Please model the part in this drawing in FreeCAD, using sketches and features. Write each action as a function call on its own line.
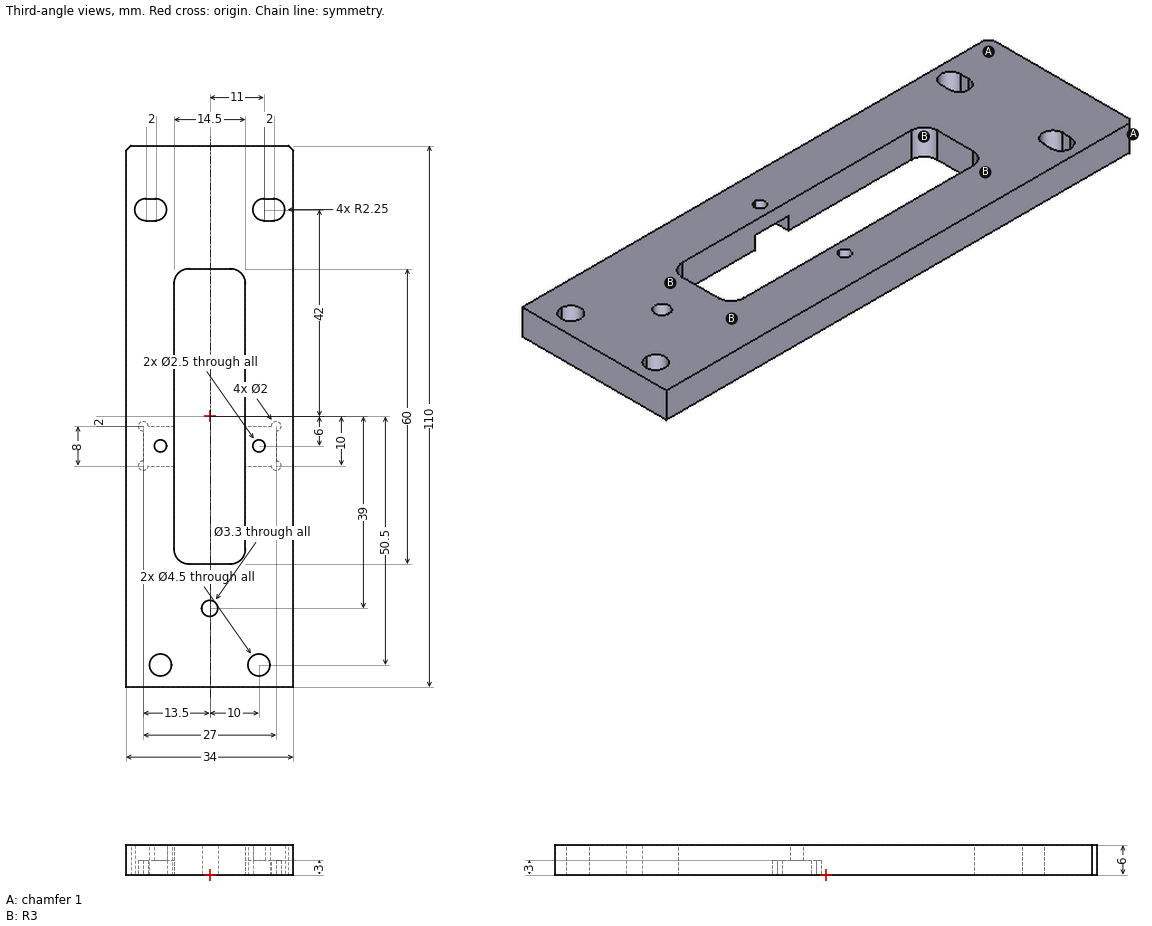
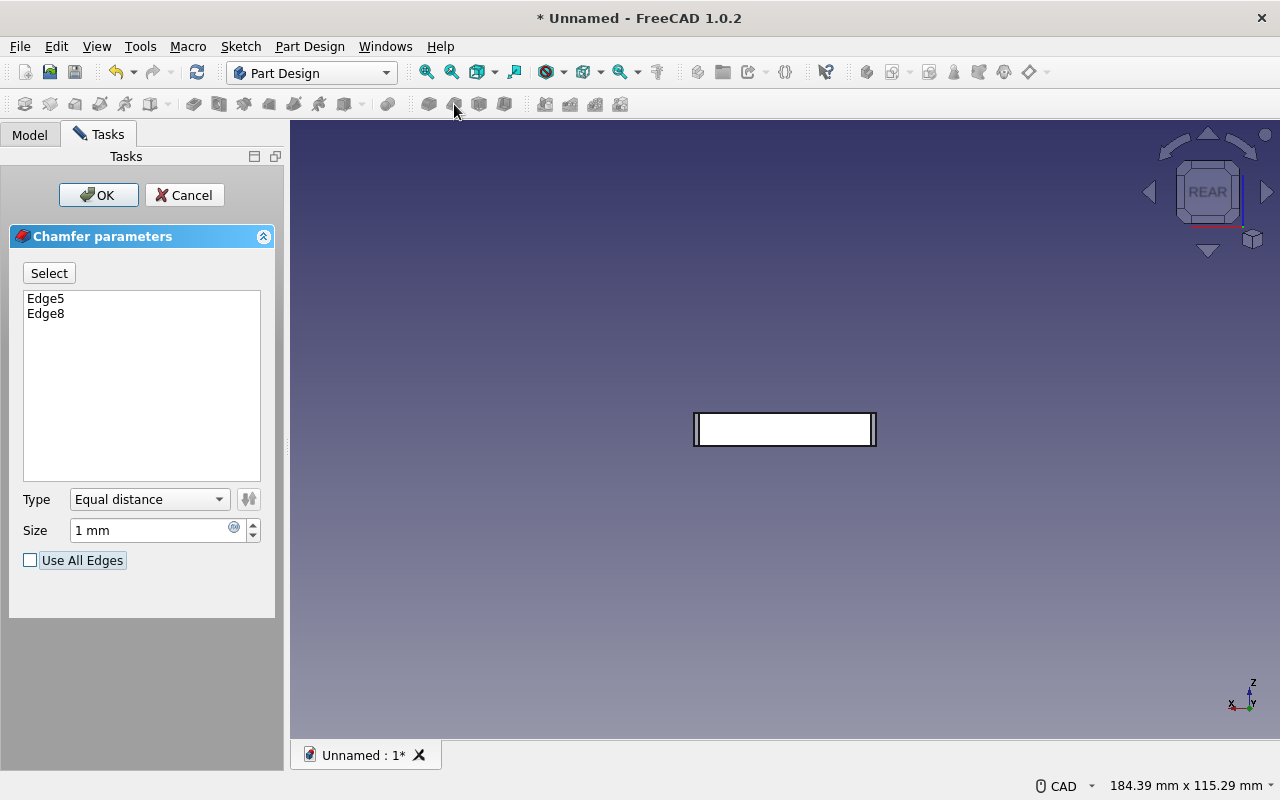
click(99, 195)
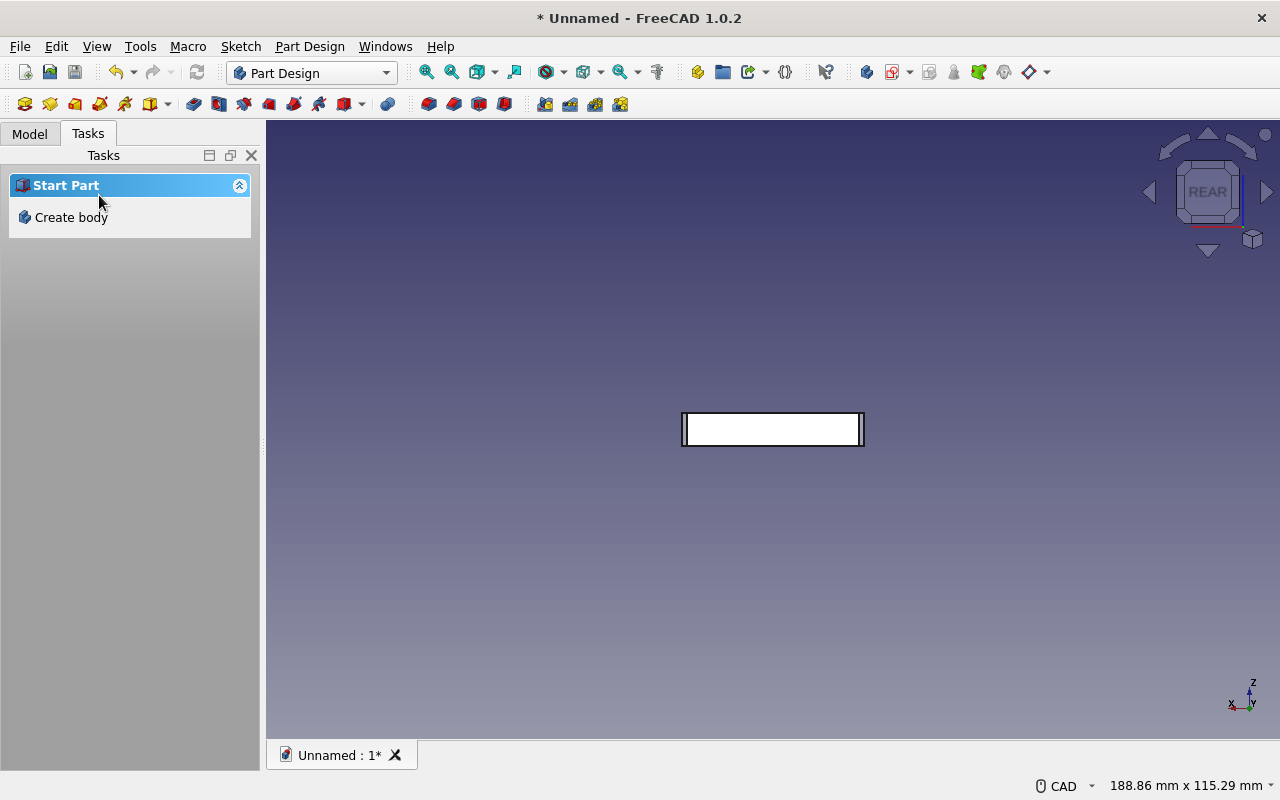
key(v)
key(f)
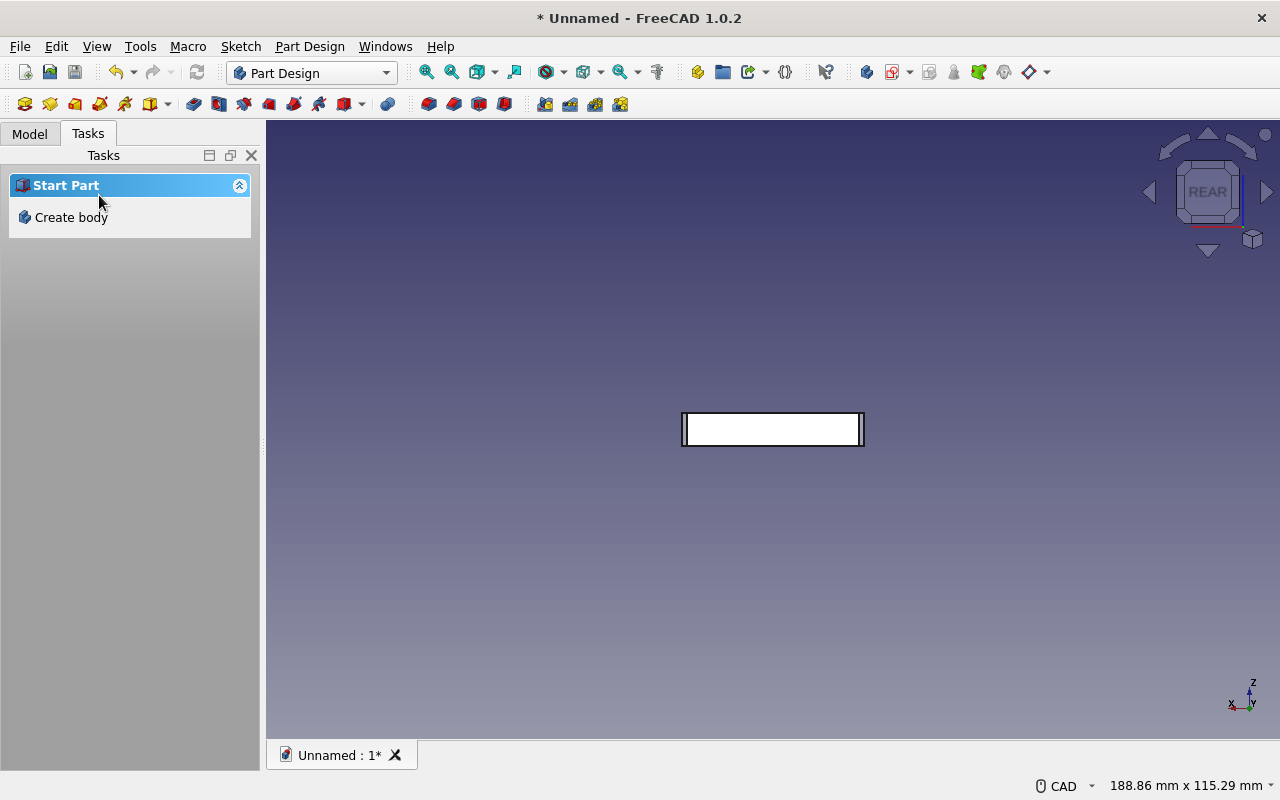
key(5)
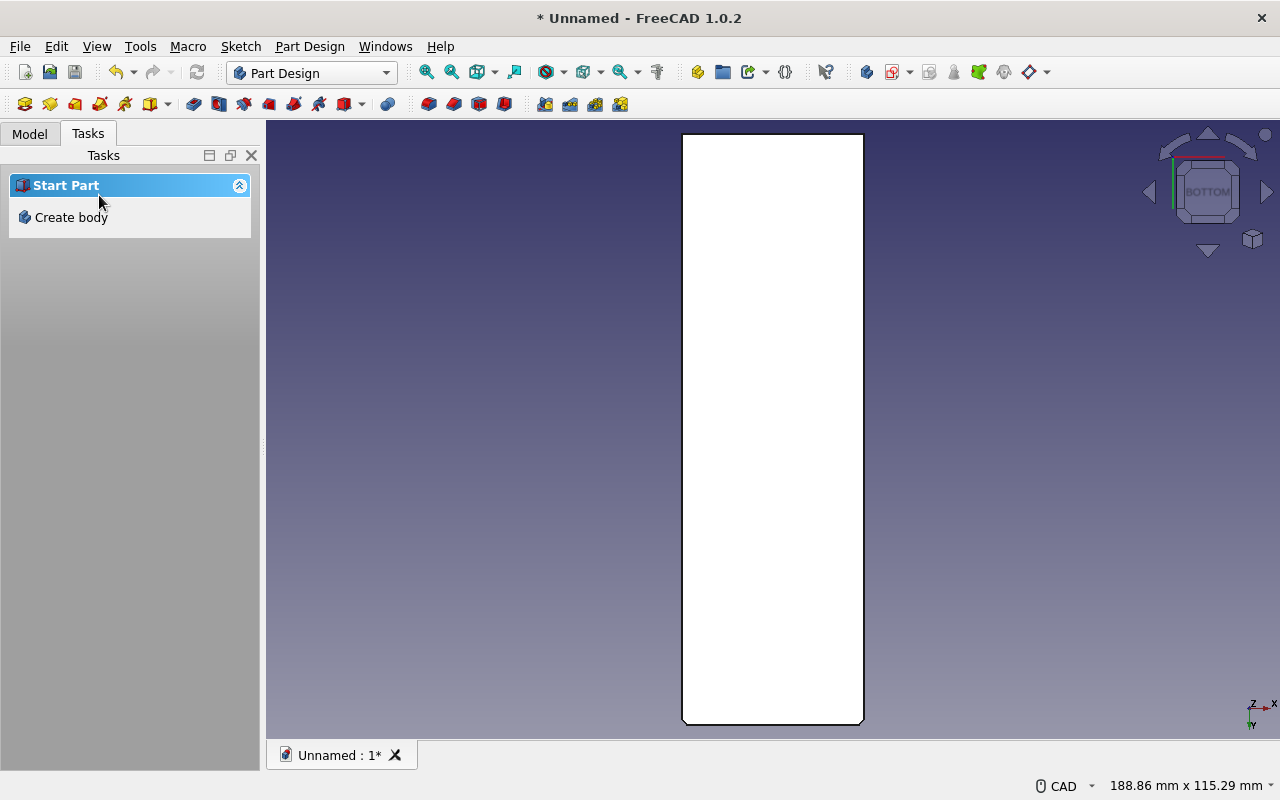
click(773, 597)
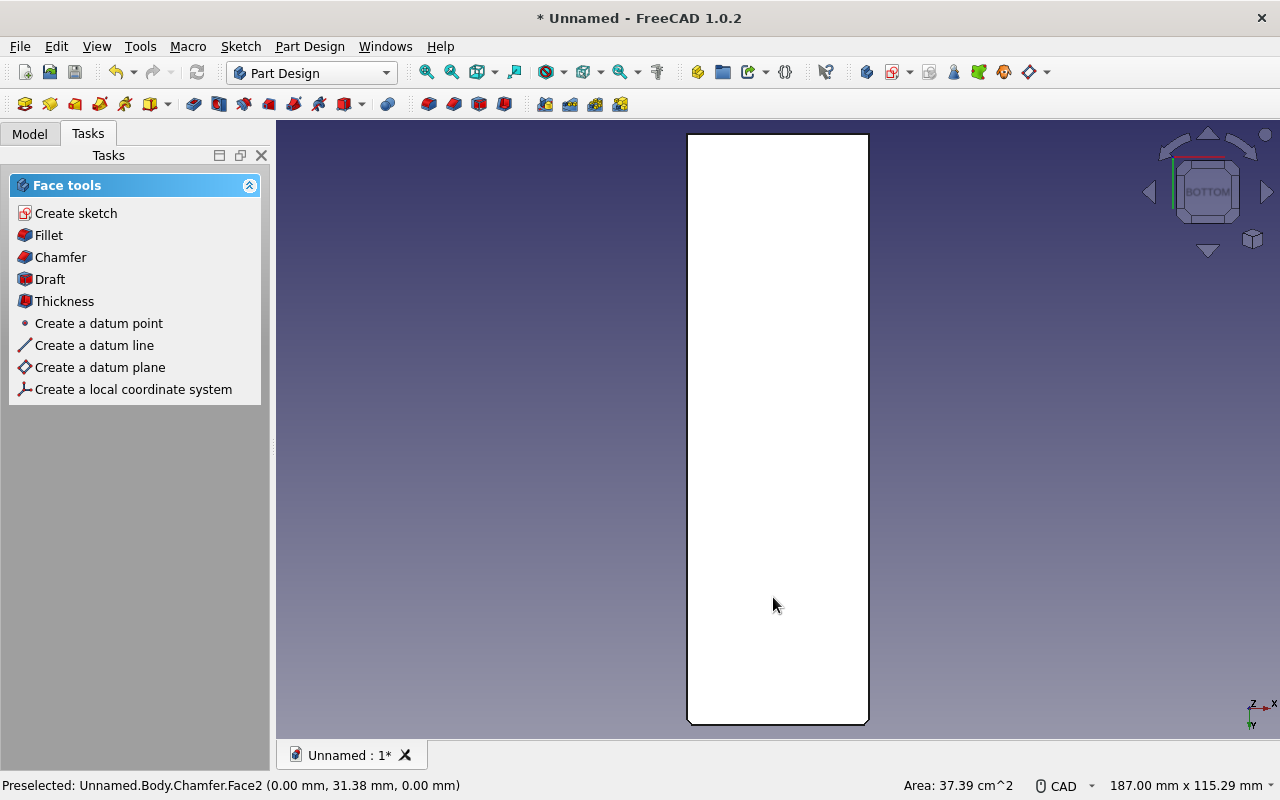
click(892, 72)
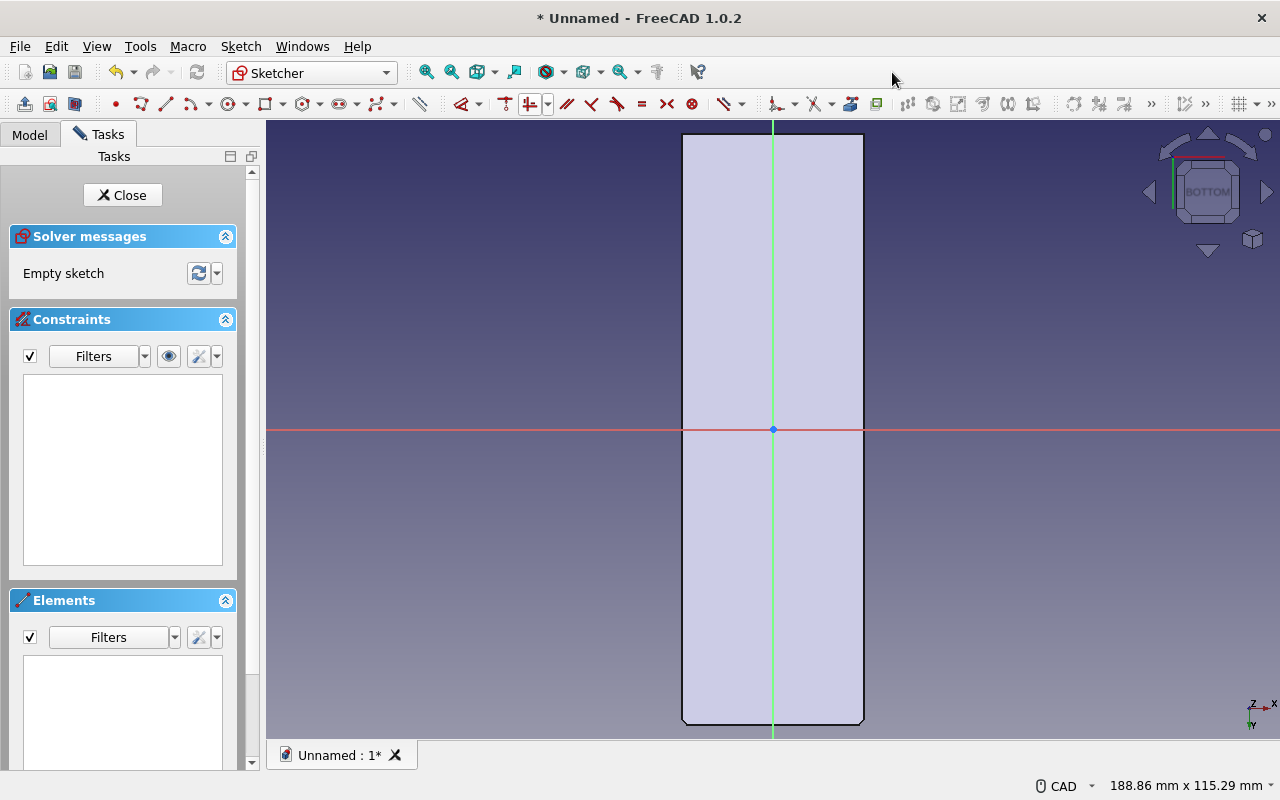
scroll(395, 711, down, 1)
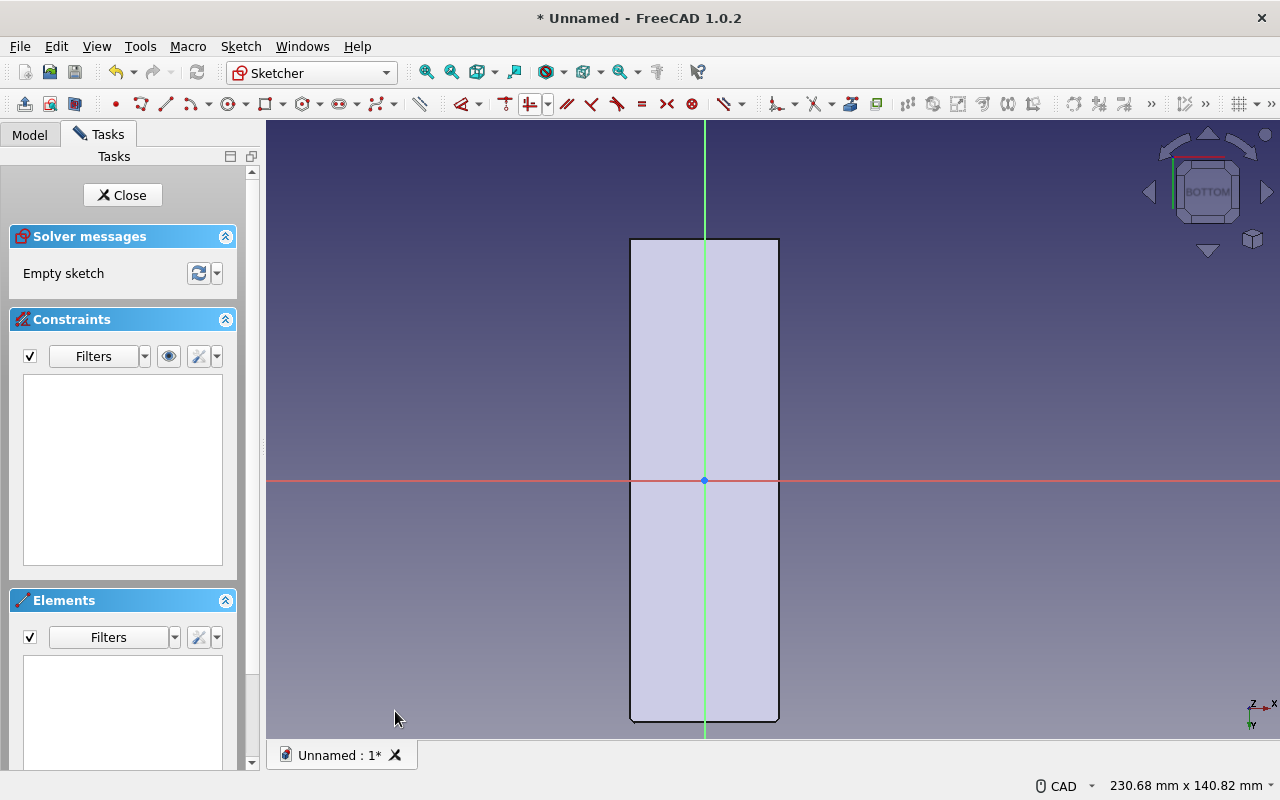
scroll(705, 286, up, 3)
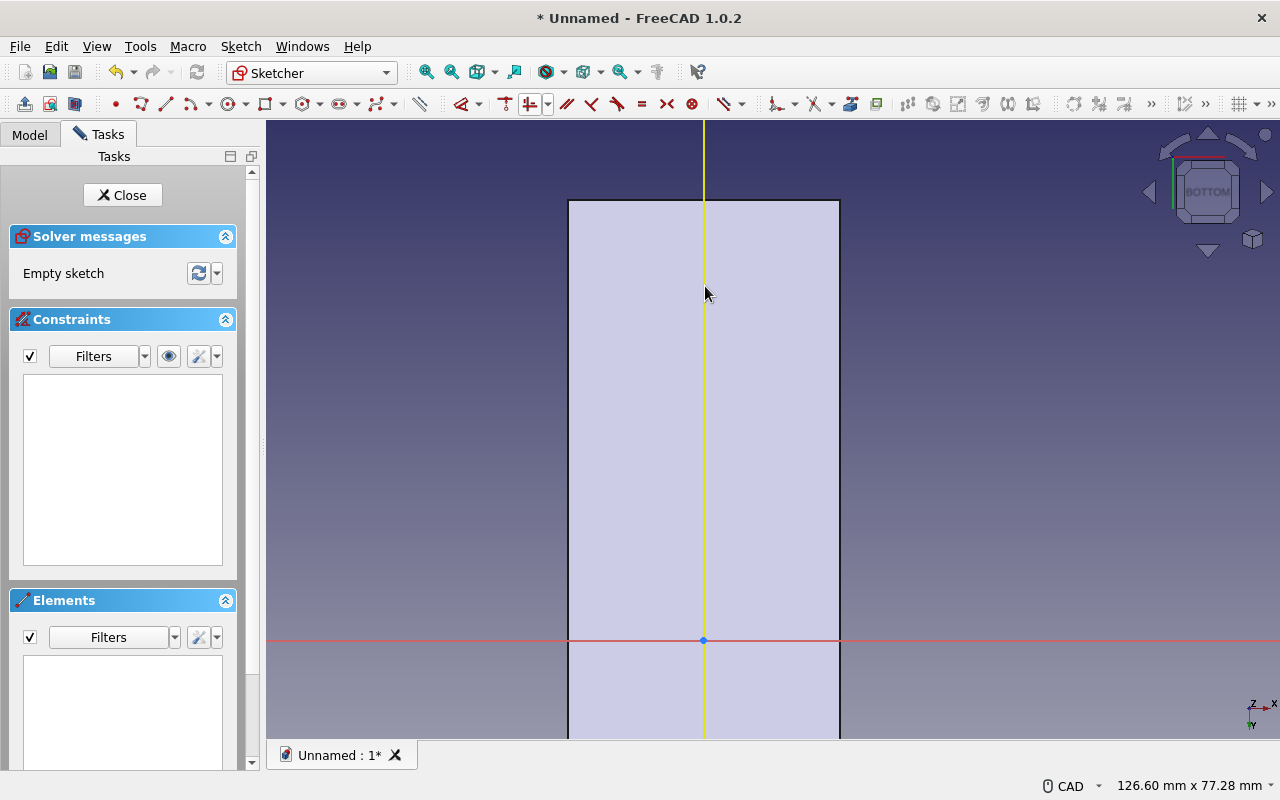
key(g)
key(c)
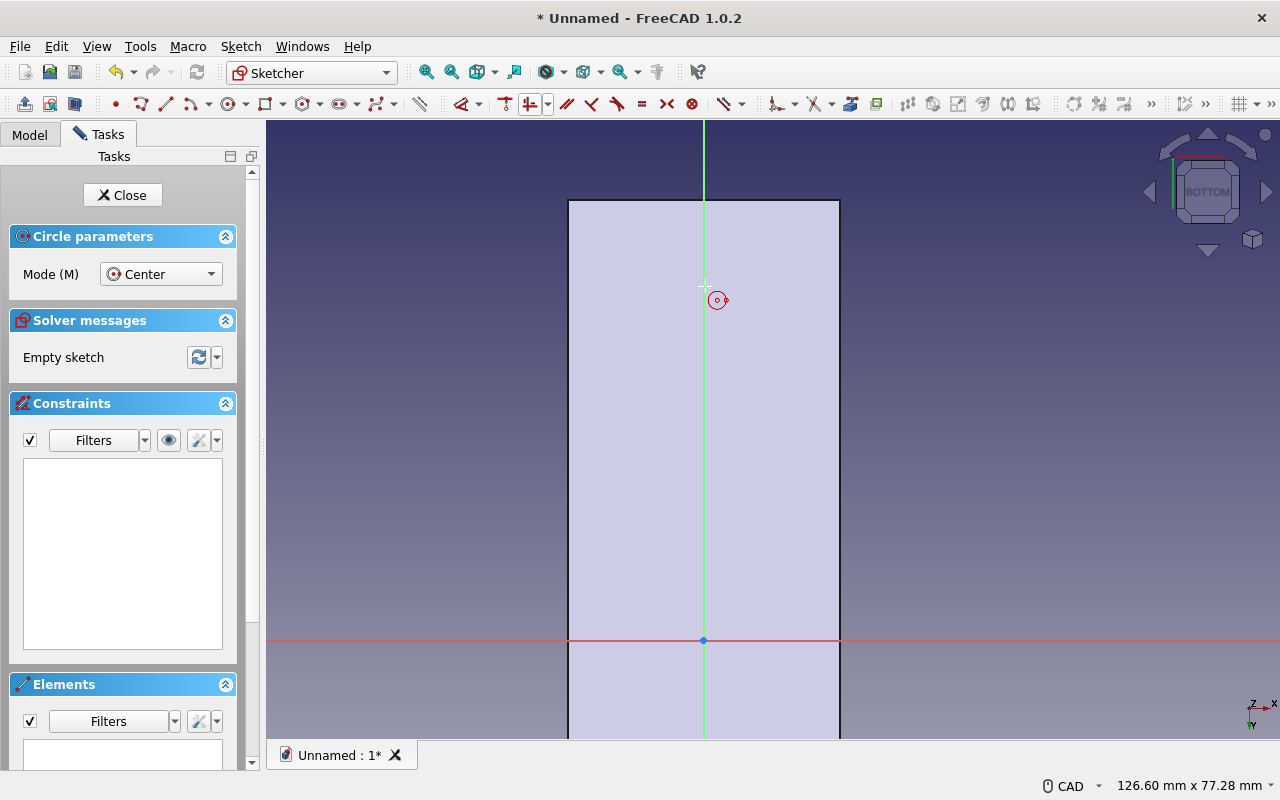
scroll(784, 236, up, 2)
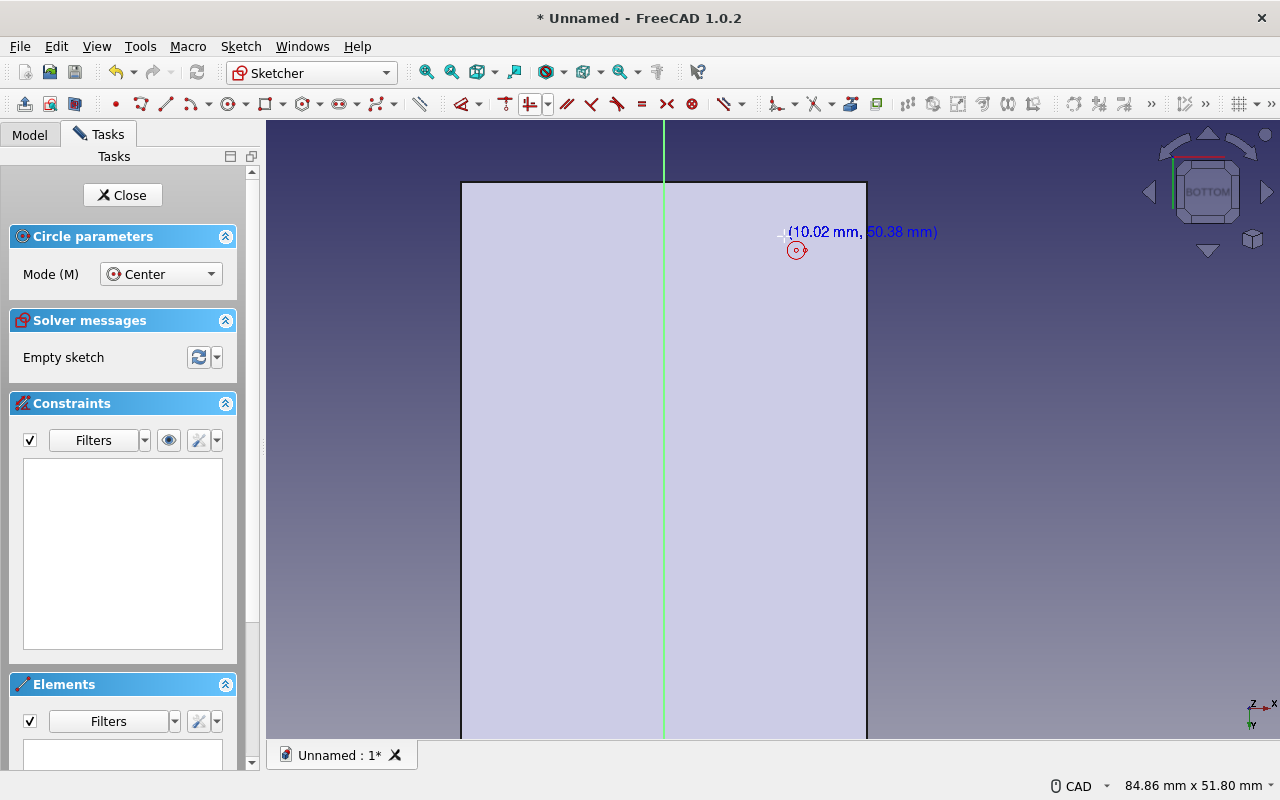
click(784, 236)
click(803, 217)